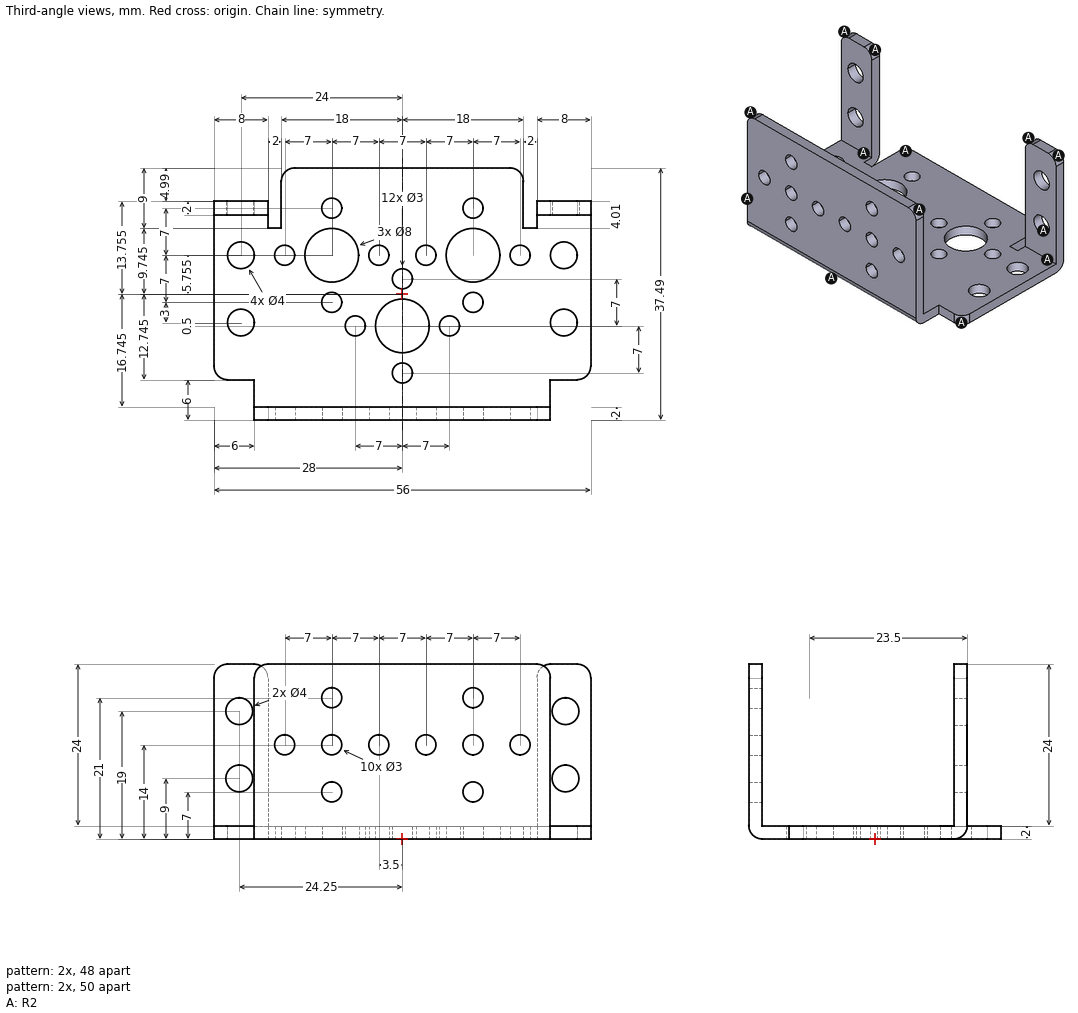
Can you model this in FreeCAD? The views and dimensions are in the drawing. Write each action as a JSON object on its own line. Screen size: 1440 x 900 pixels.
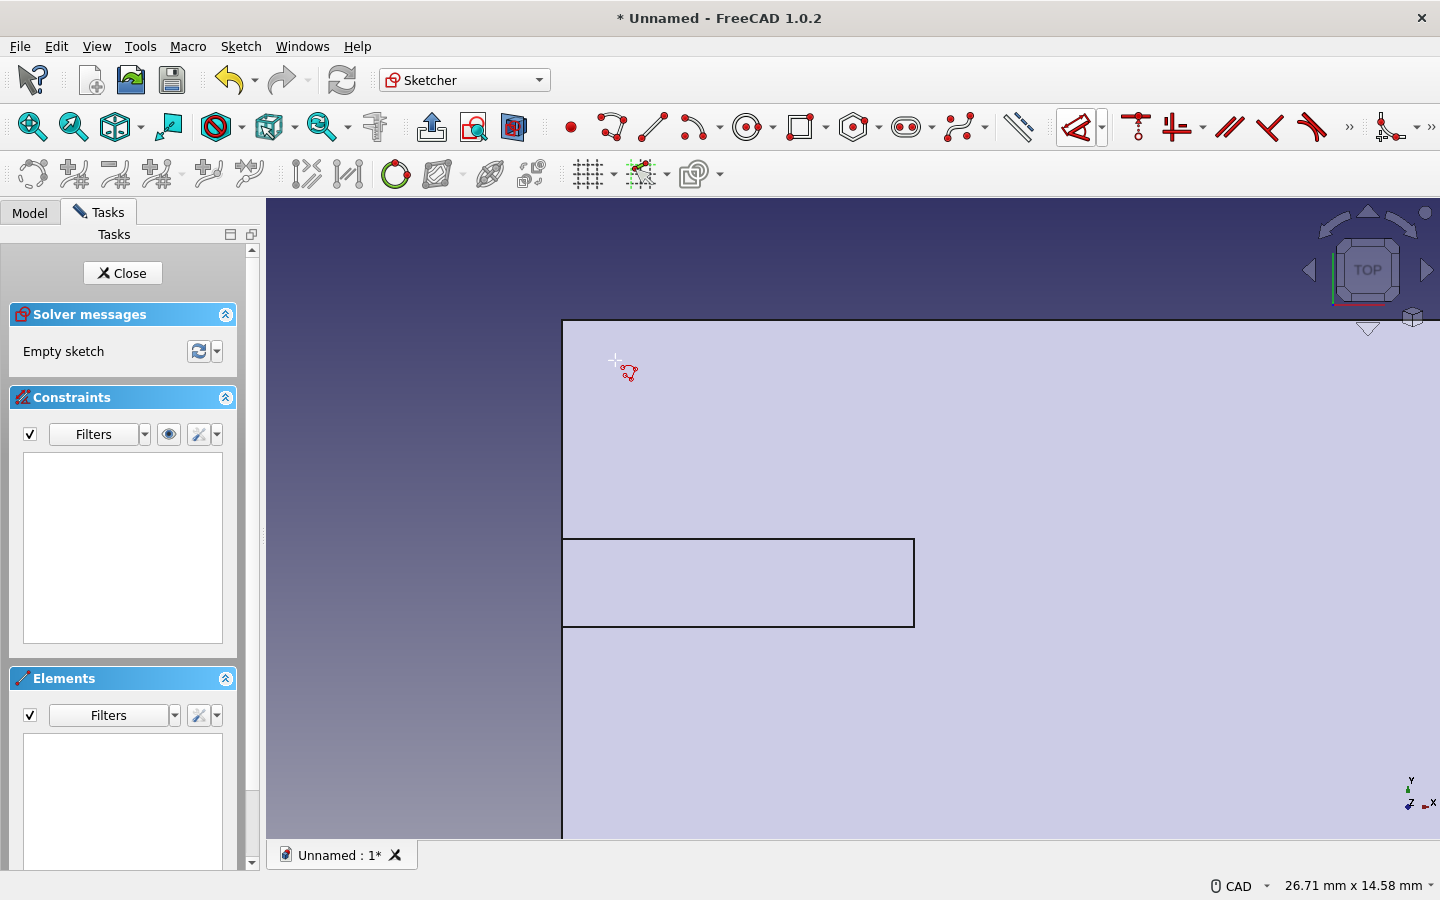
{"action": "left_click", "coordinate": [1001, 716]}
{"action": "left_click", "coordinate": [1001, 320]}
{"action": "left_click", "coordinate": [562, 320]}
{"action": "left_click", "coordinate": [562, 539]}
{"action": "left_click", "coordinate": [914, 539]}
{"action": "left_click", "coordinate": [914, 716]}
{"action": "left_click", "coordinate": [1001, 717]}
{"action": "key", "text": "Escape"}
{"action": "key", "text": "Escape"}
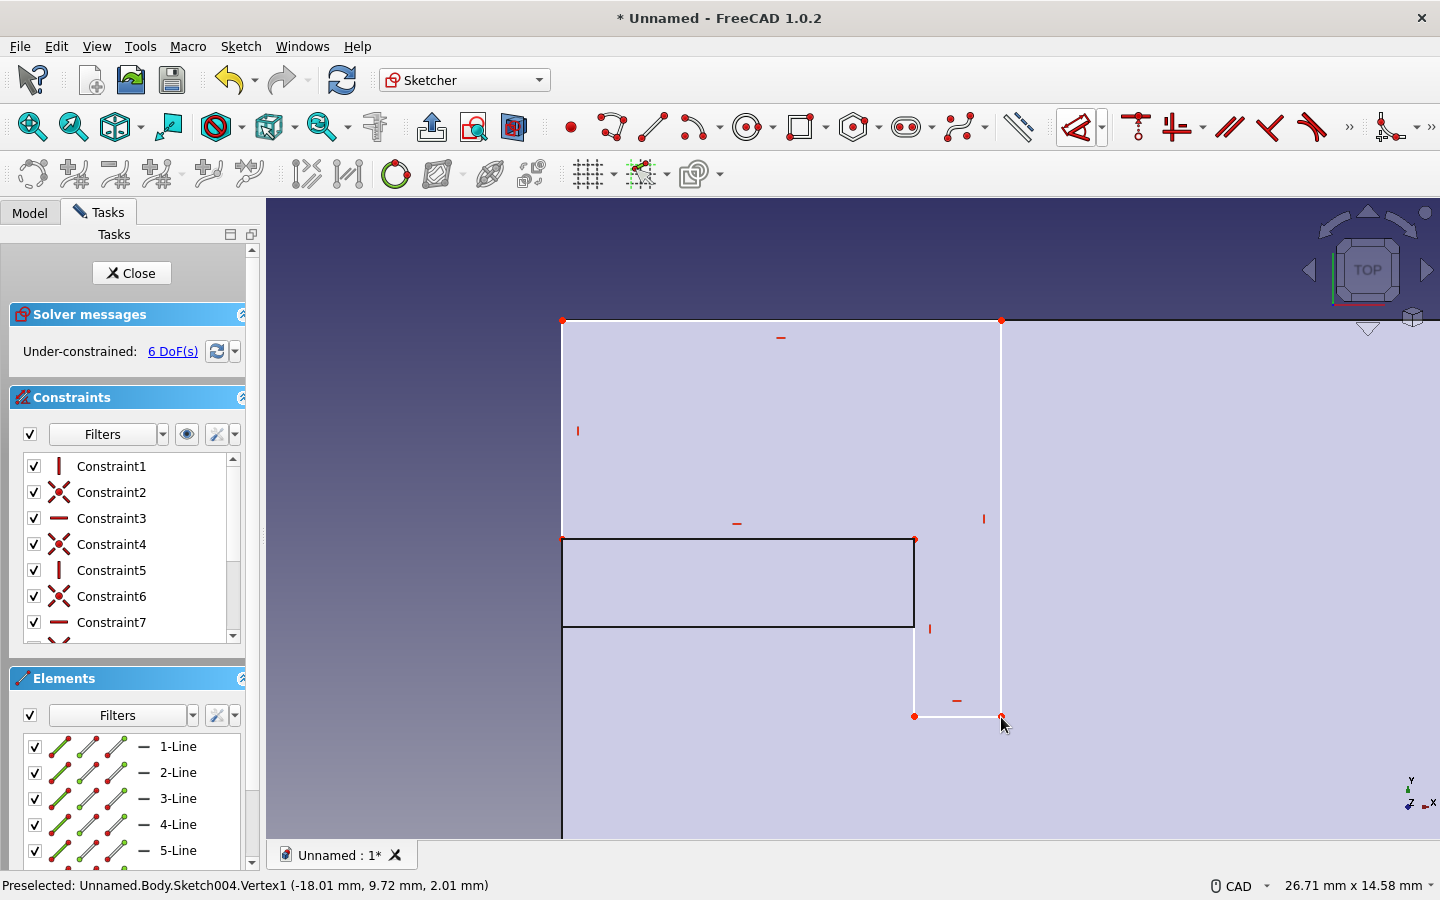
{"action": "left_click", "coordinate": [1001, 598]}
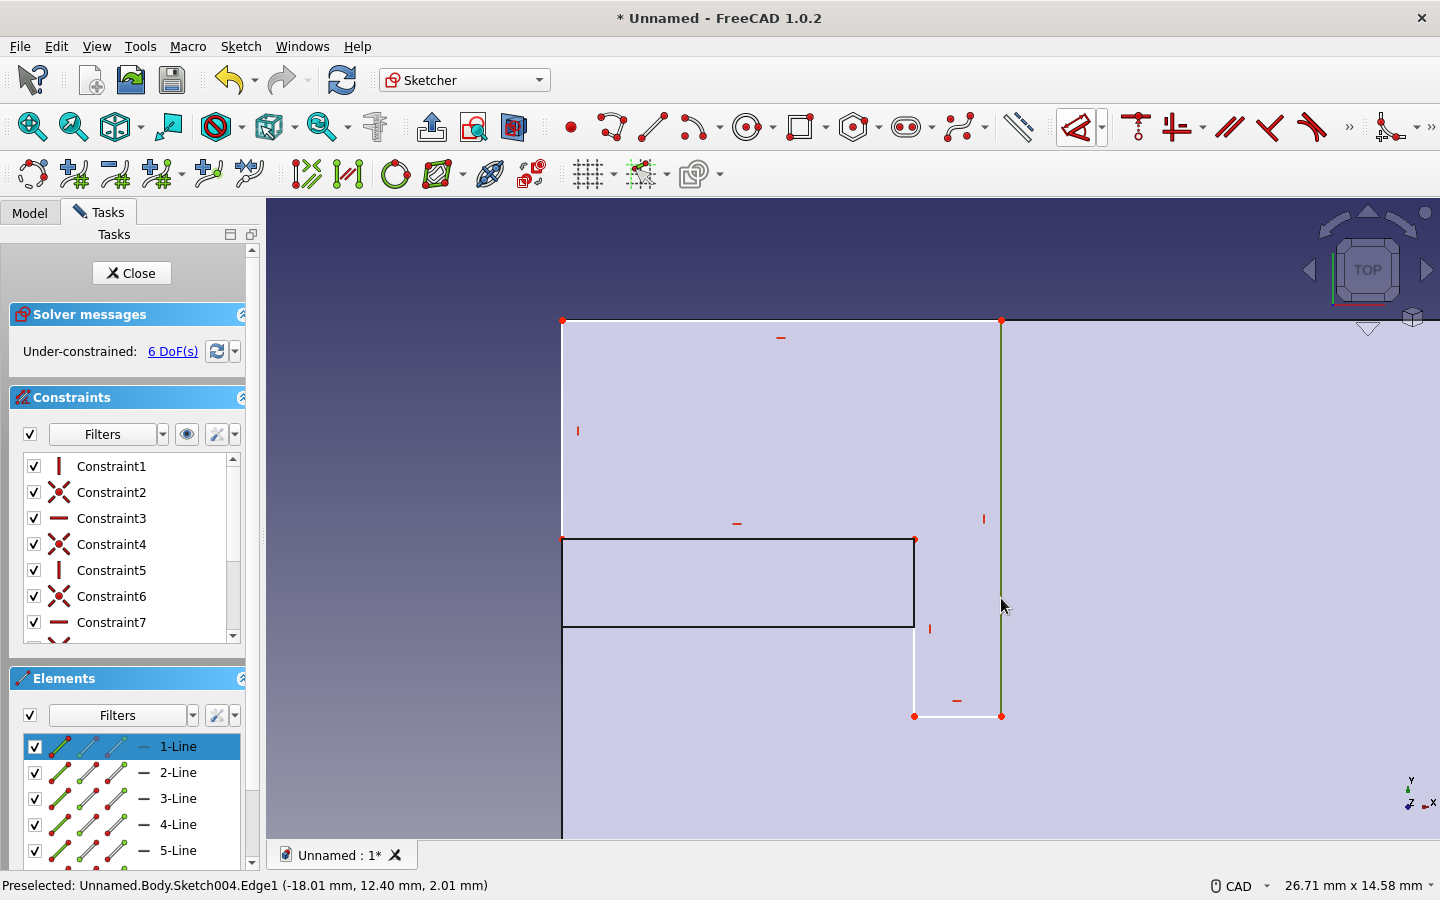
{"action": "key", "text": "i"}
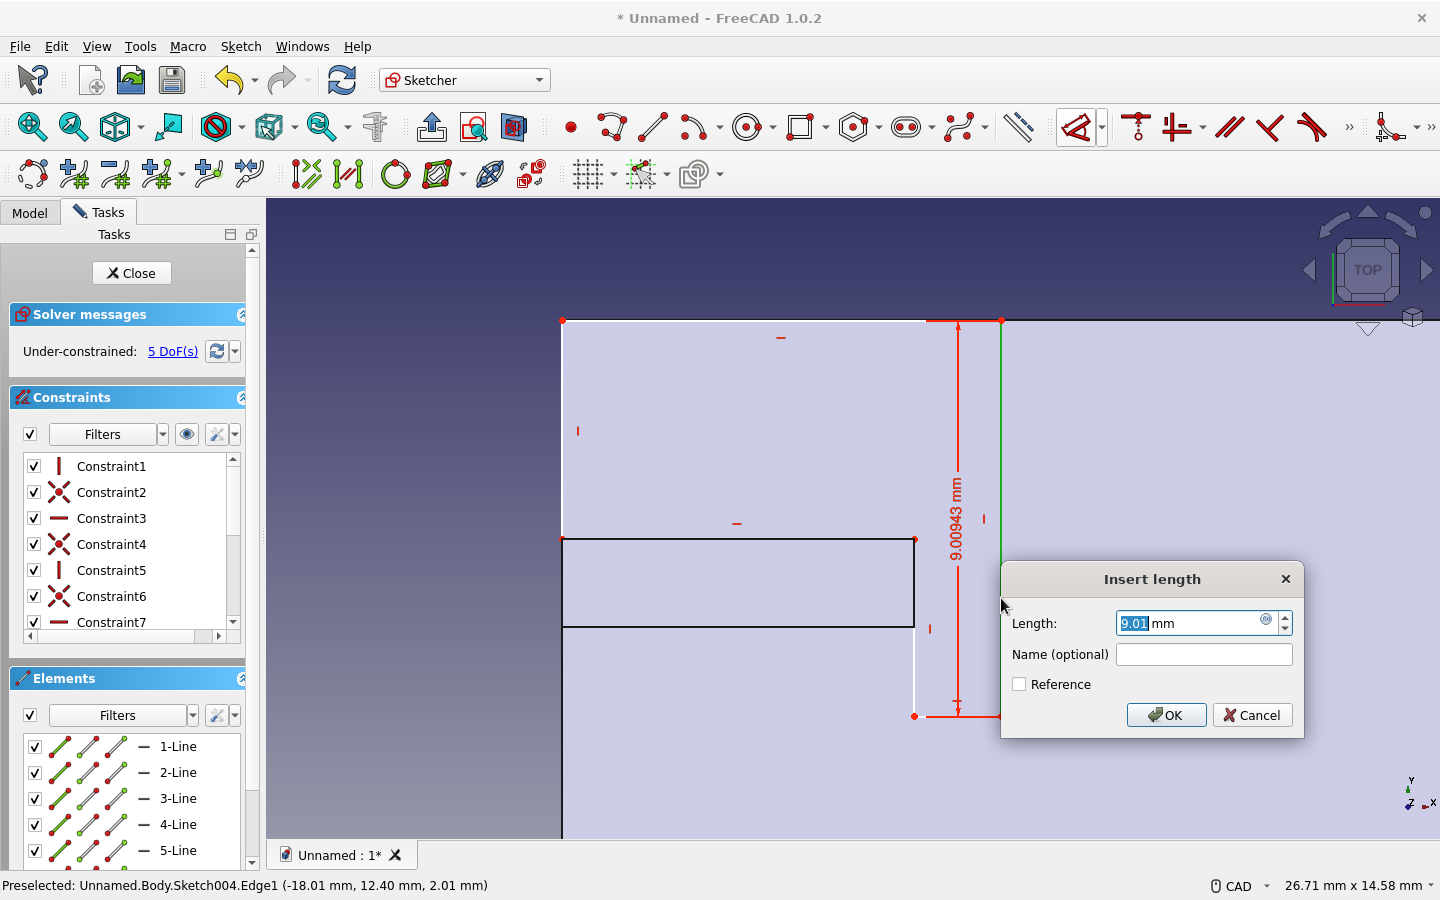
{"action": "type", "text": "9"}
{"action": "key", "text": "Return"}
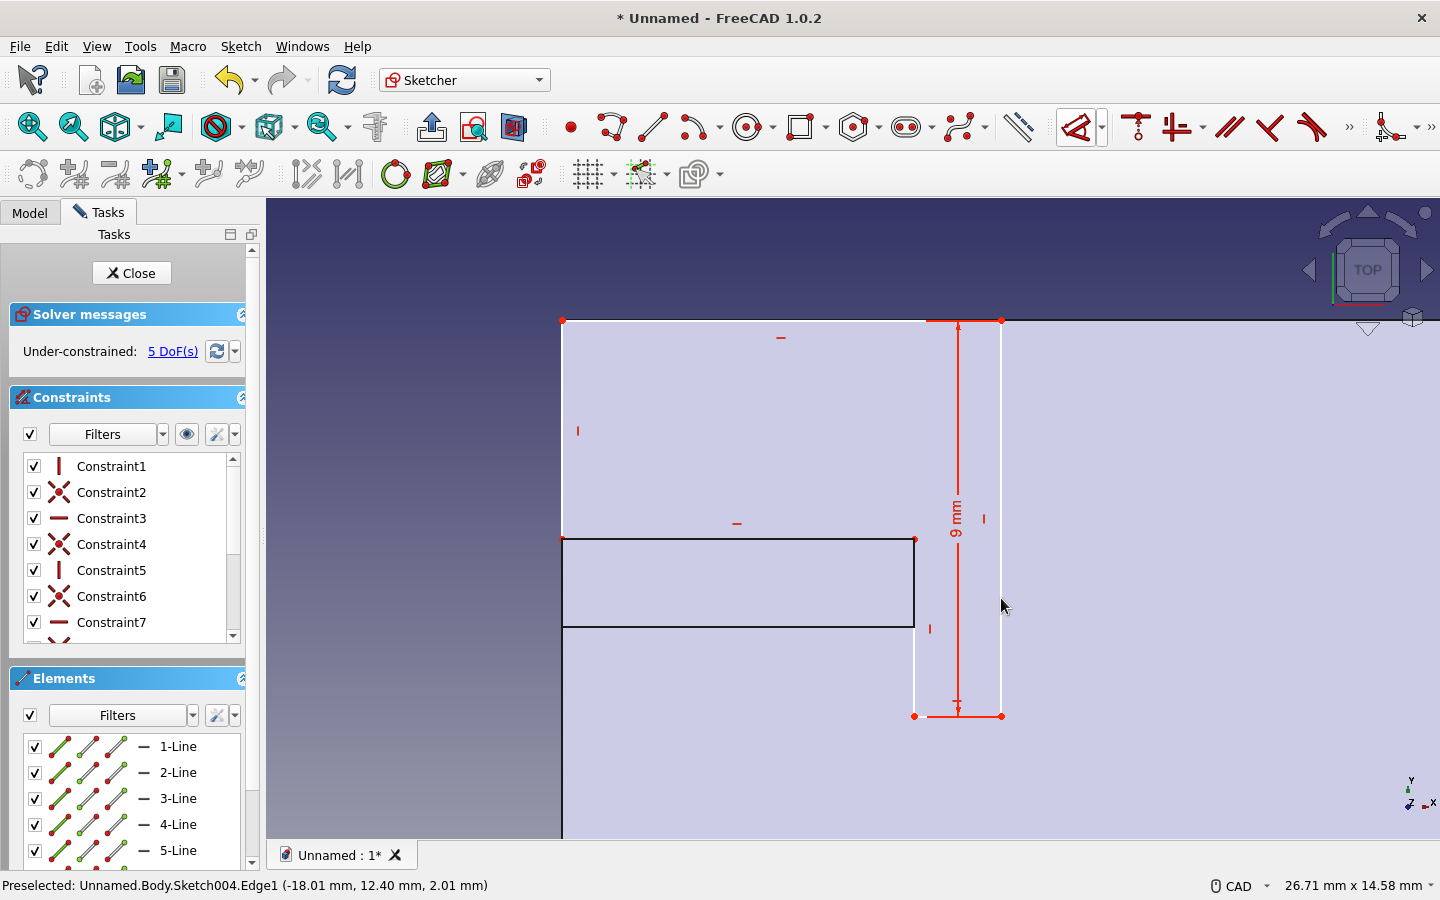
{"action": "left_click", "coordinate": [668, 540]}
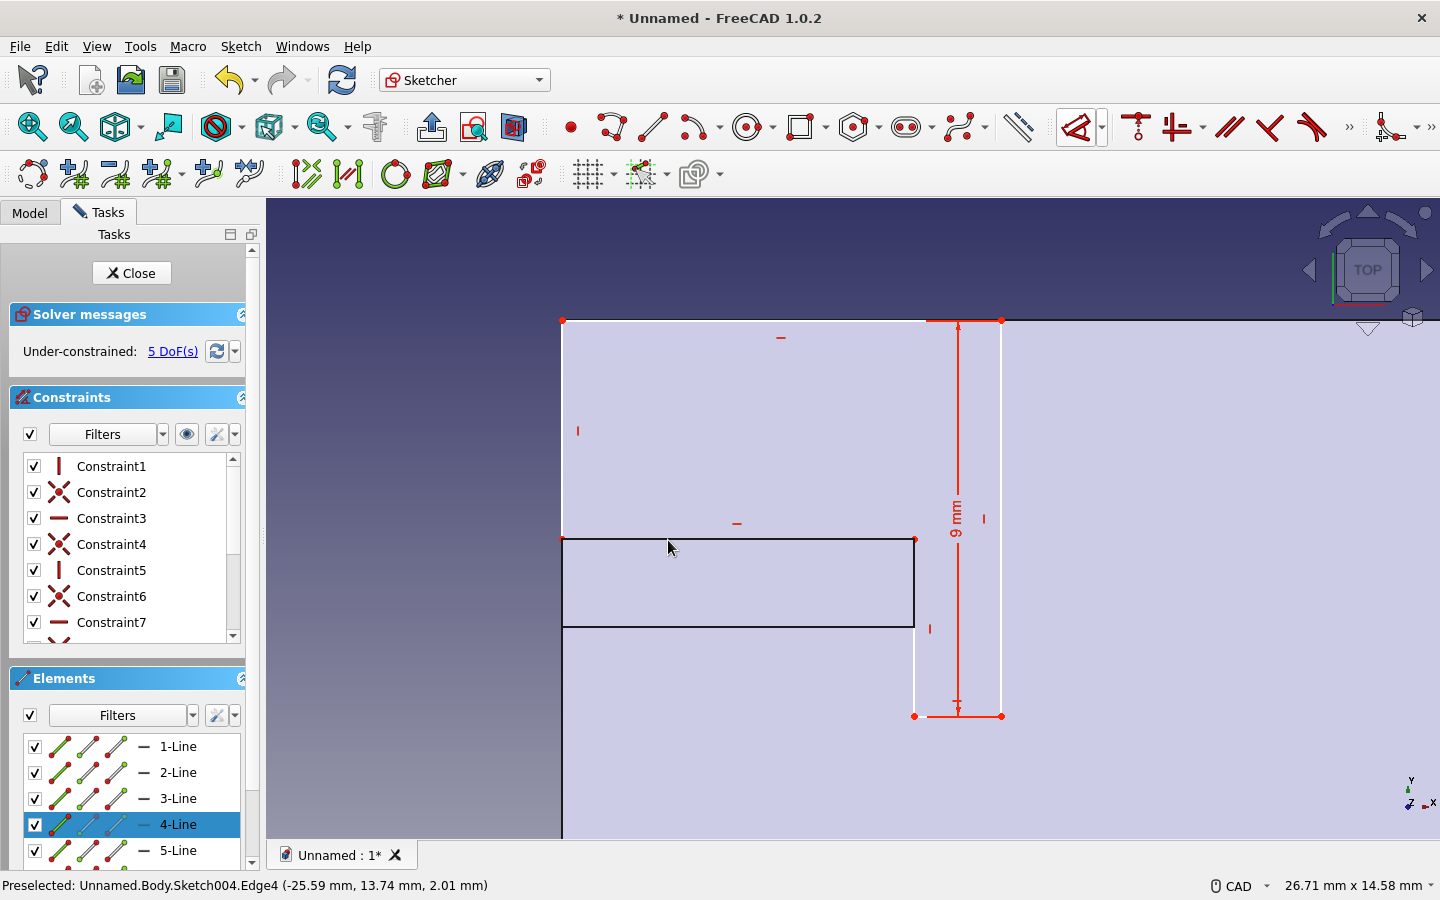
{"action": "key", "text": "l"}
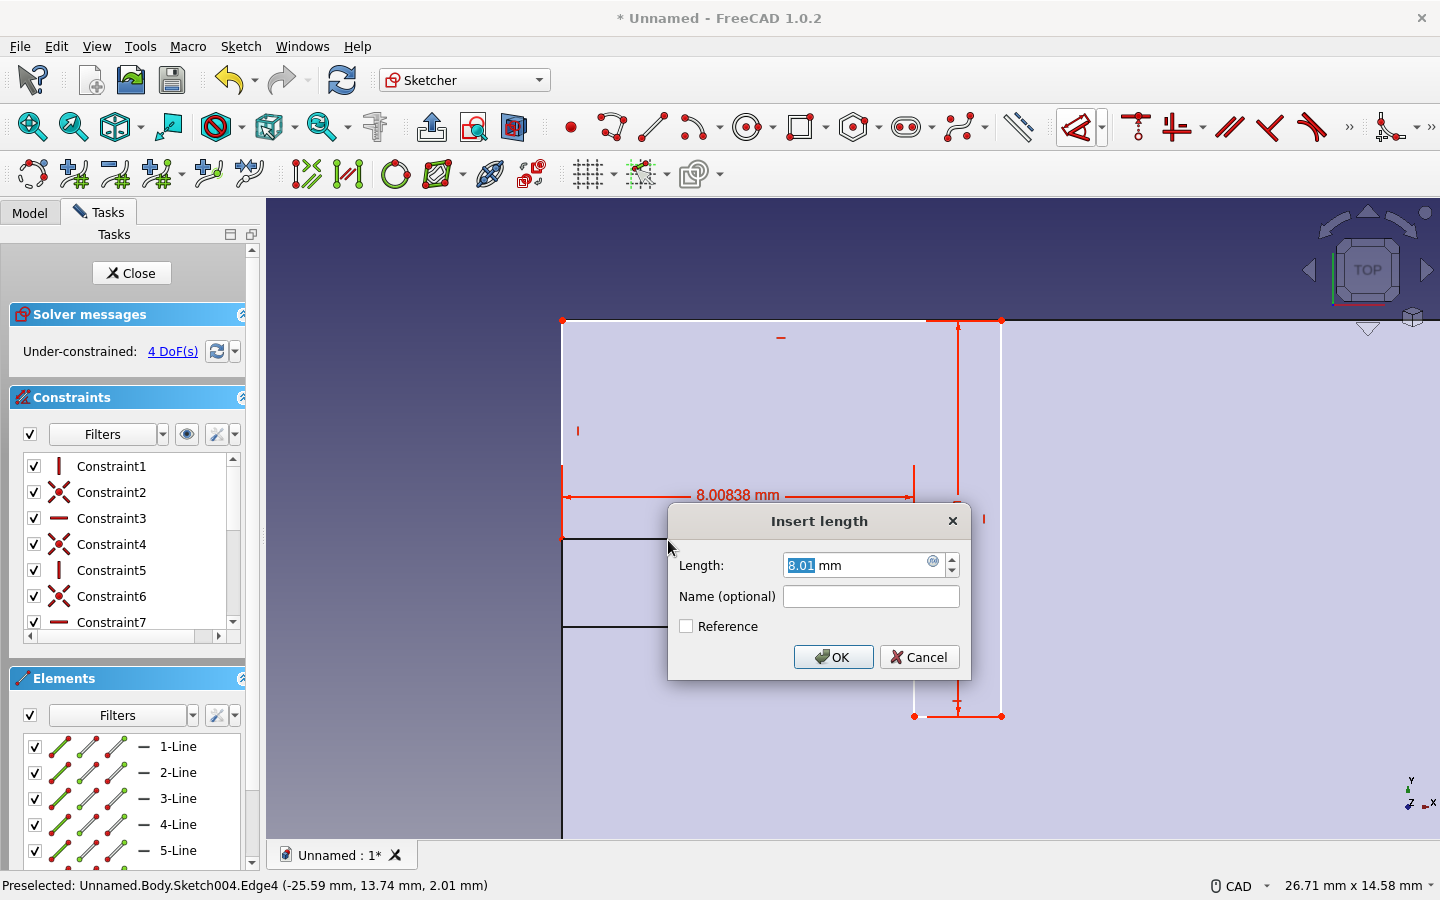
{"action": "type", "text": "8"}
{"action": "key", "text": "Return"}